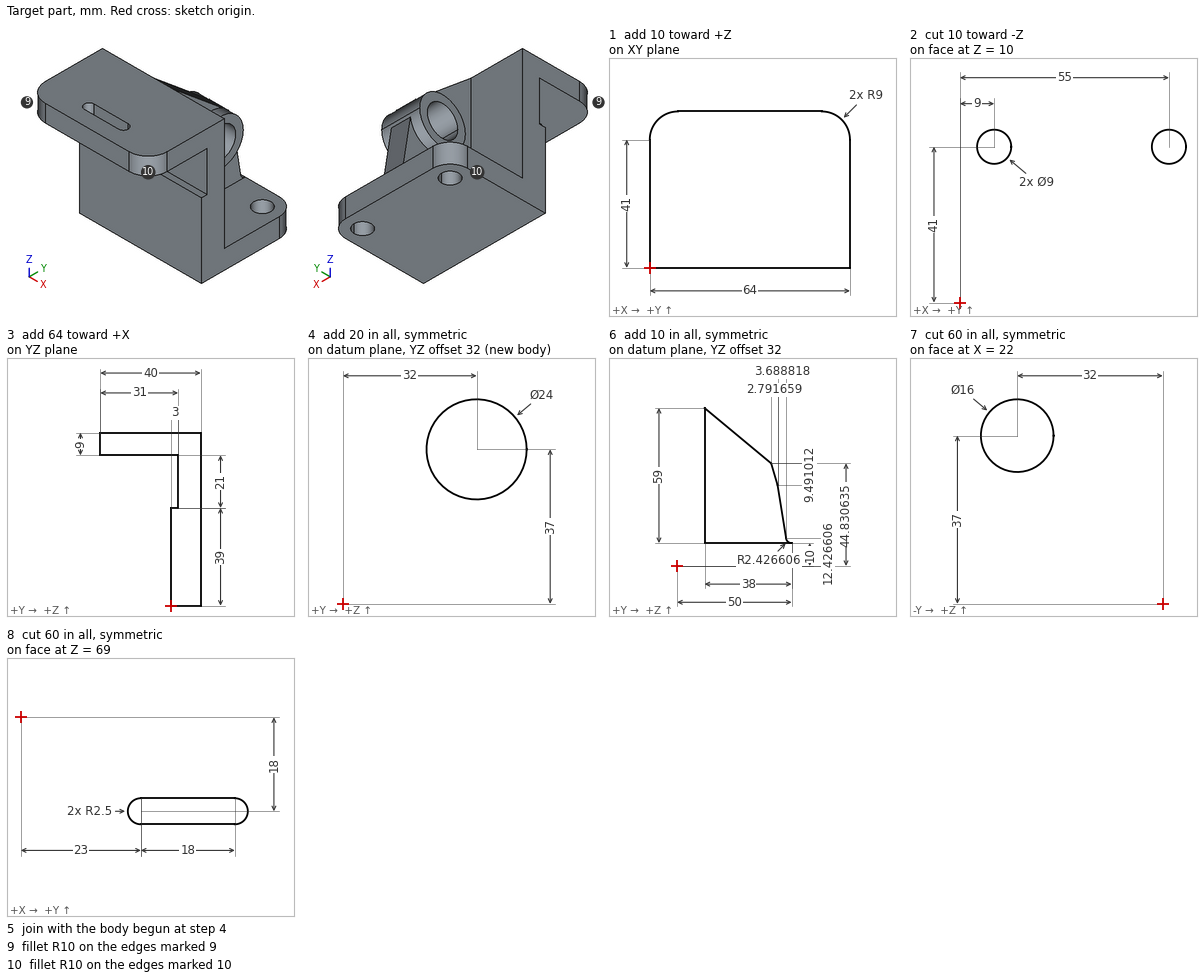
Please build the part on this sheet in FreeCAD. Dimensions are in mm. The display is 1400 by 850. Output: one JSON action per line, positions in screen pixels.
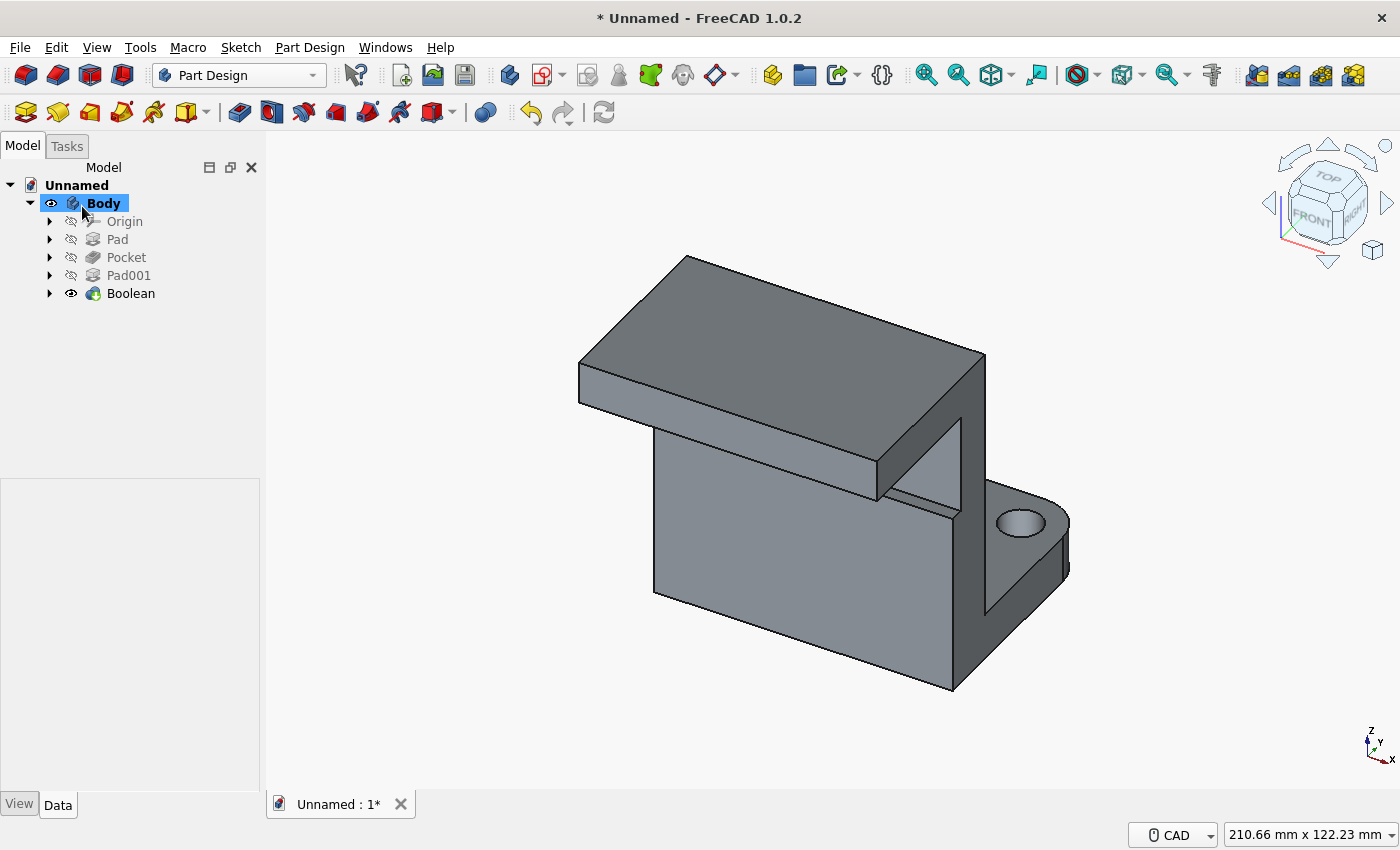
{"action": "left_click", "coordinate": [50, 221]}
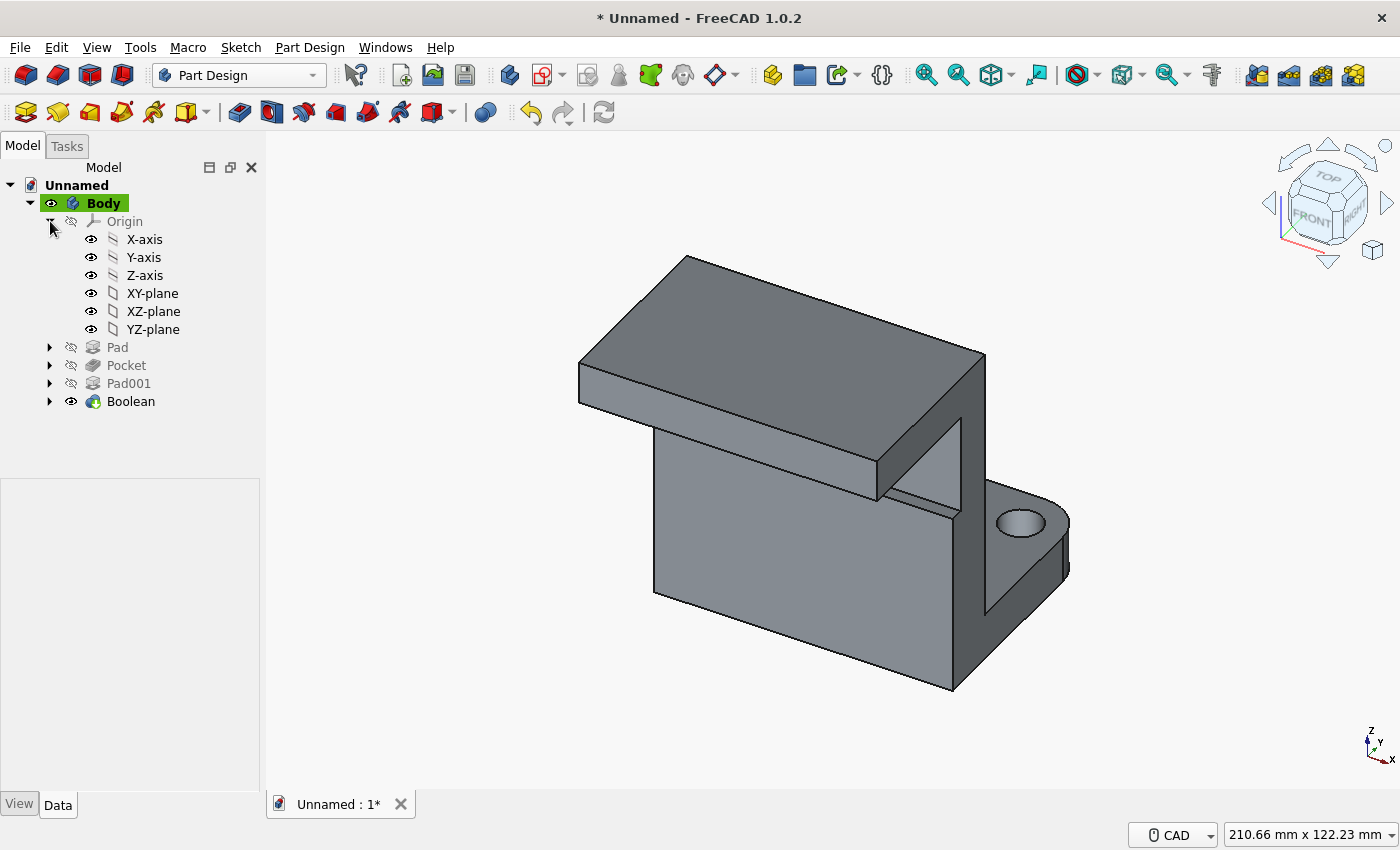
{"action": "left_click", "coordinate": [136, 329]}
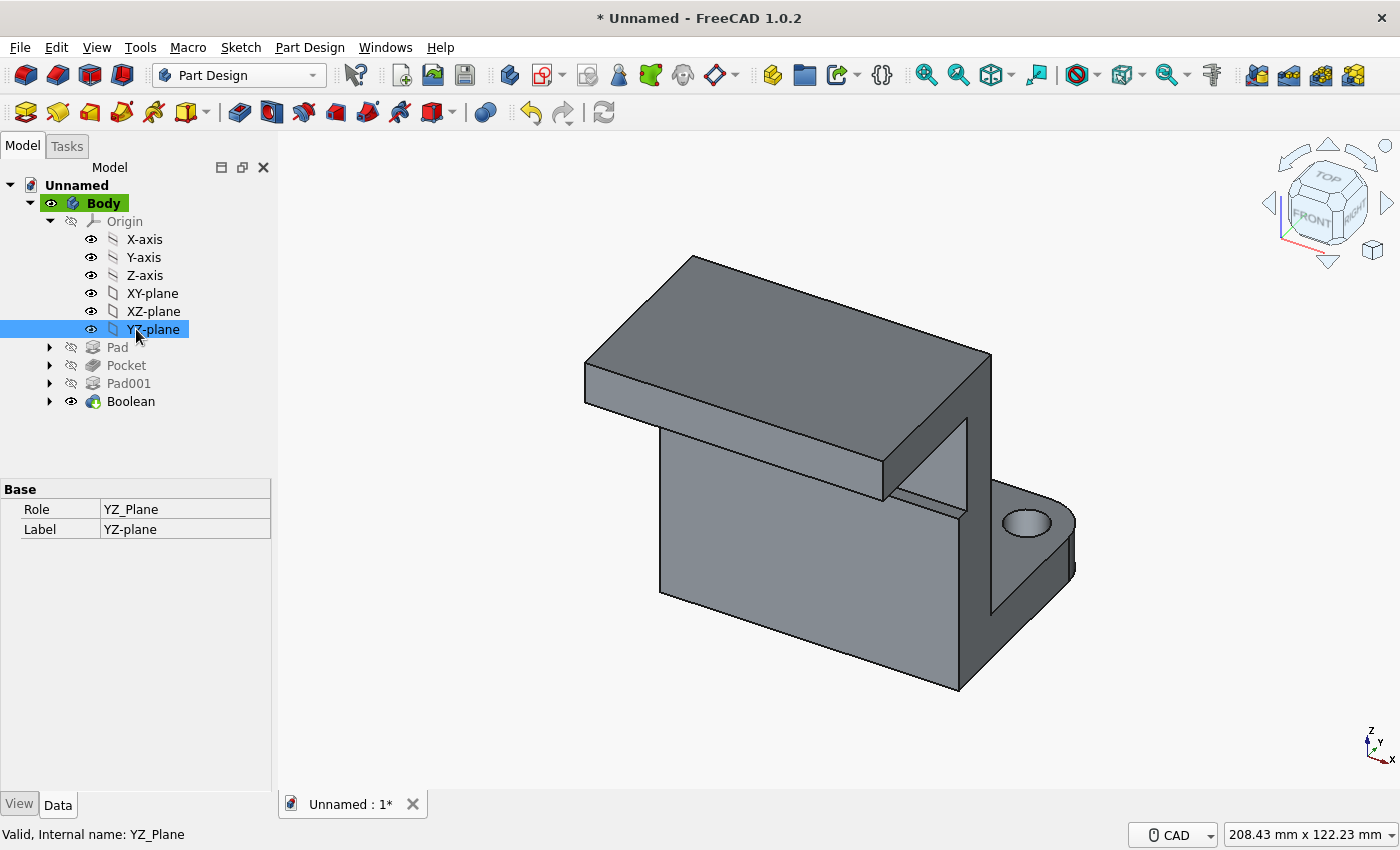
{"action": "left_click", "coordinate": [716, 76]}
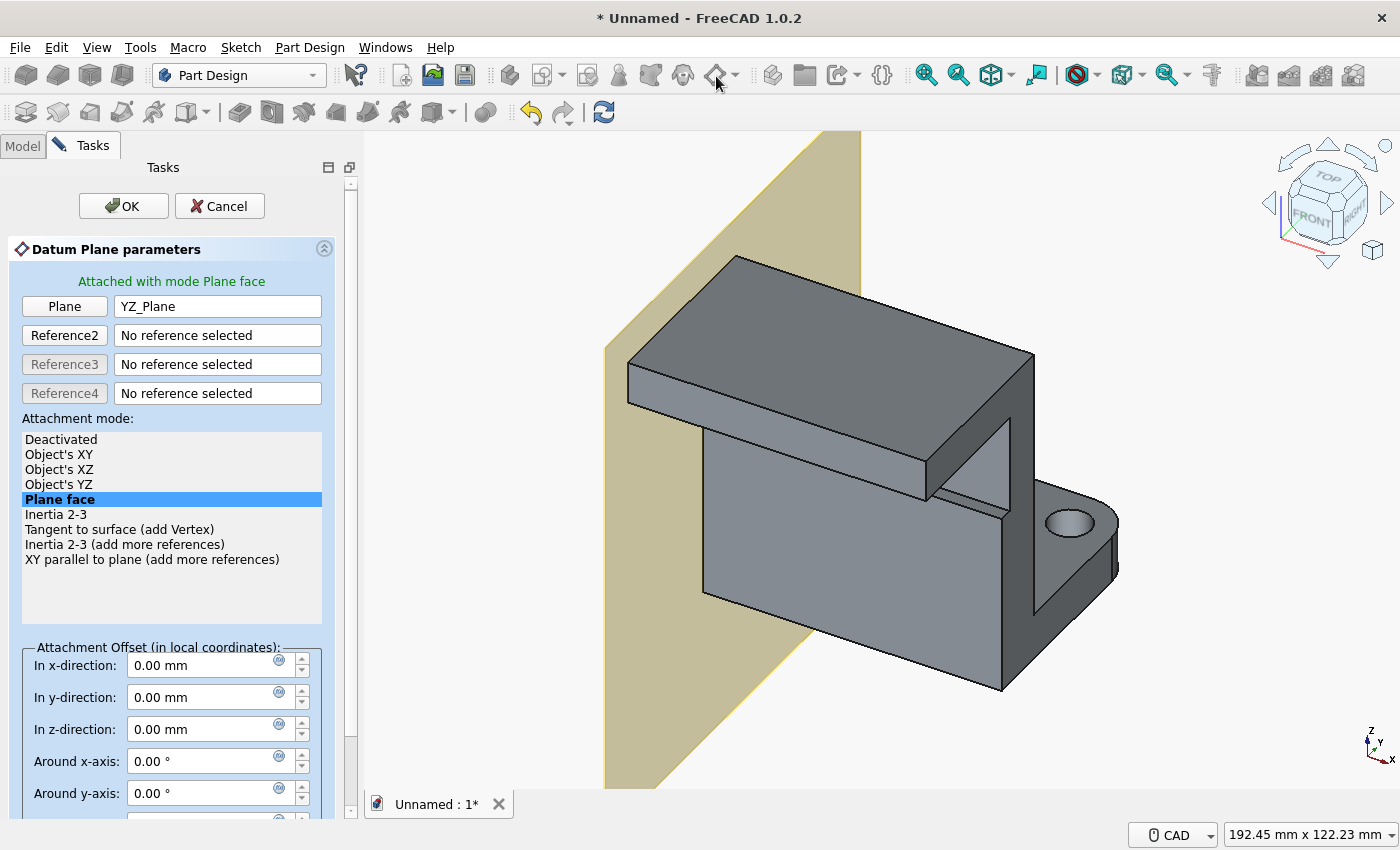
{"action": "triple_click", "coordinate": [210, 729]}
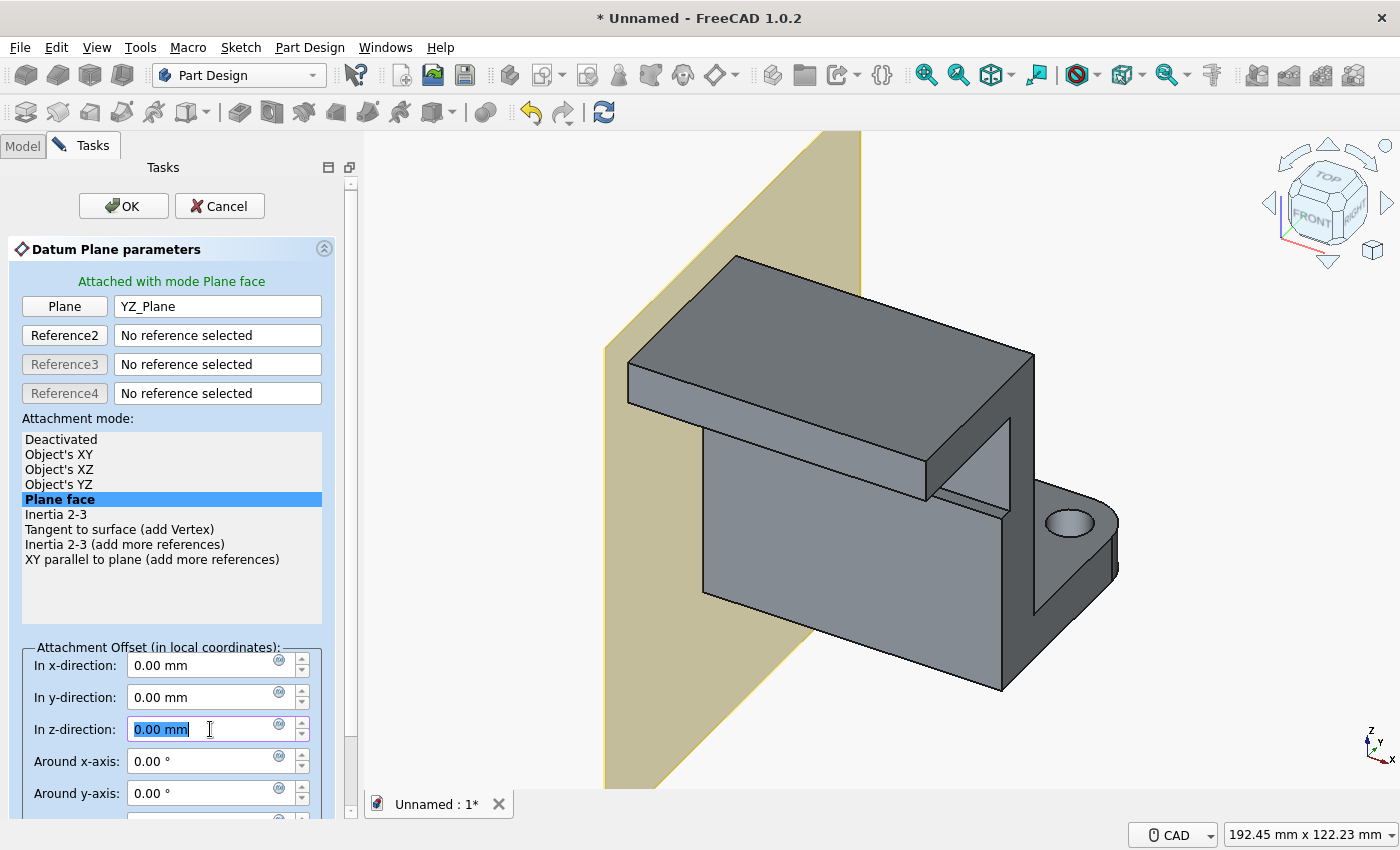
{"action": "type", "text": "32"}
{"action": "key", "text": "Tab"}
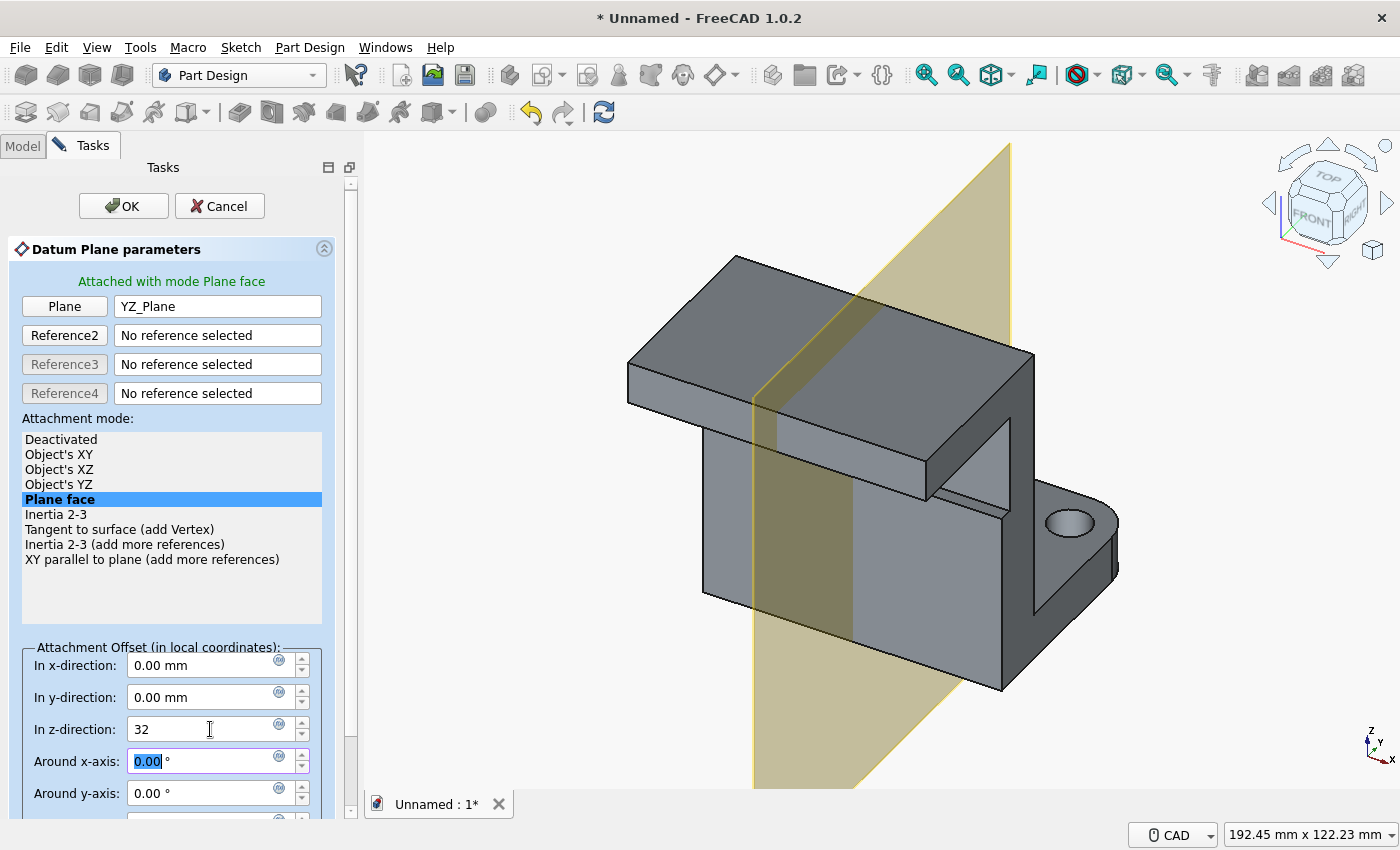
{"action": "left_click", "coordinate": [124, 206]}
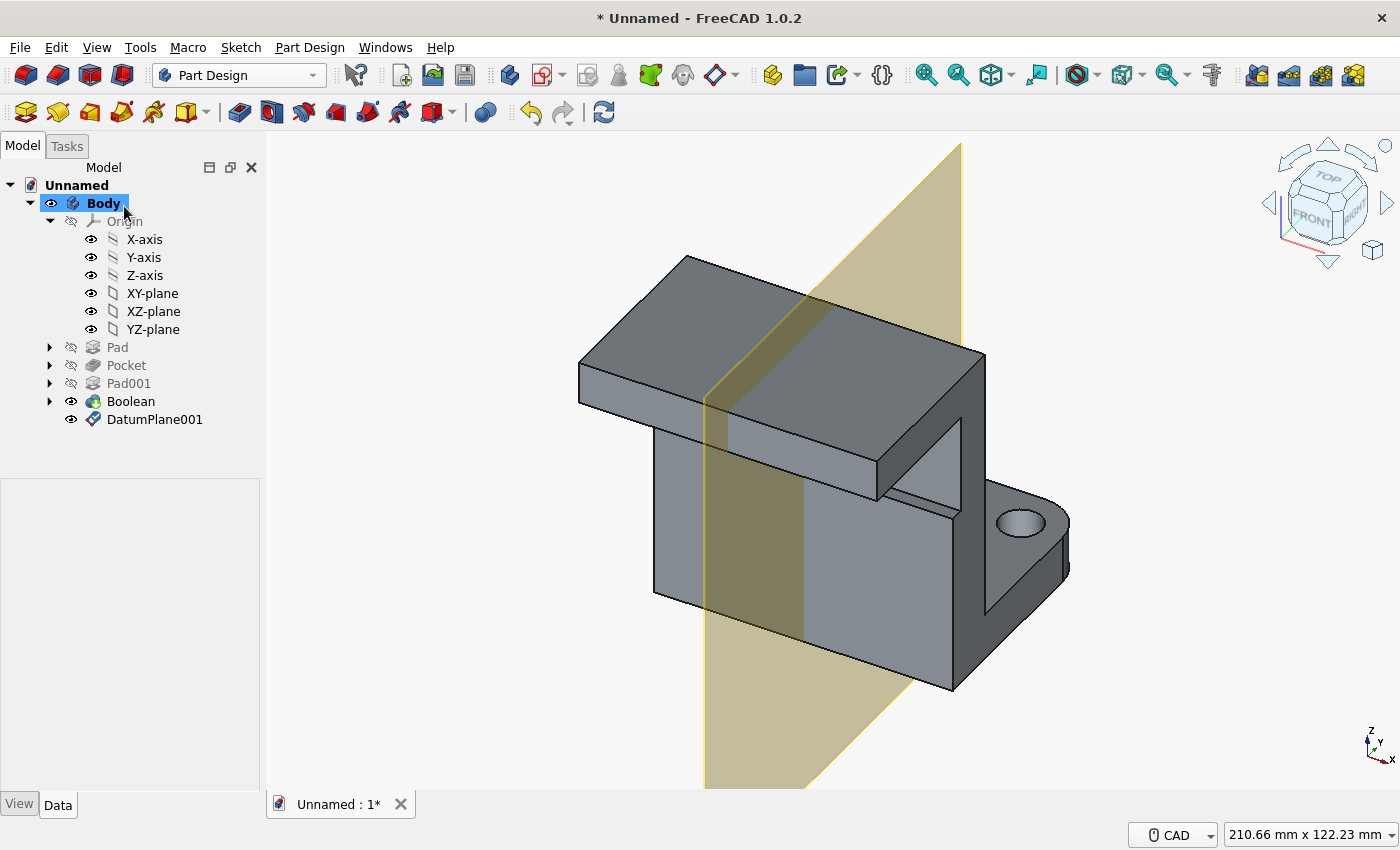
{"action": "left_click", "coordinate": [116, 419]}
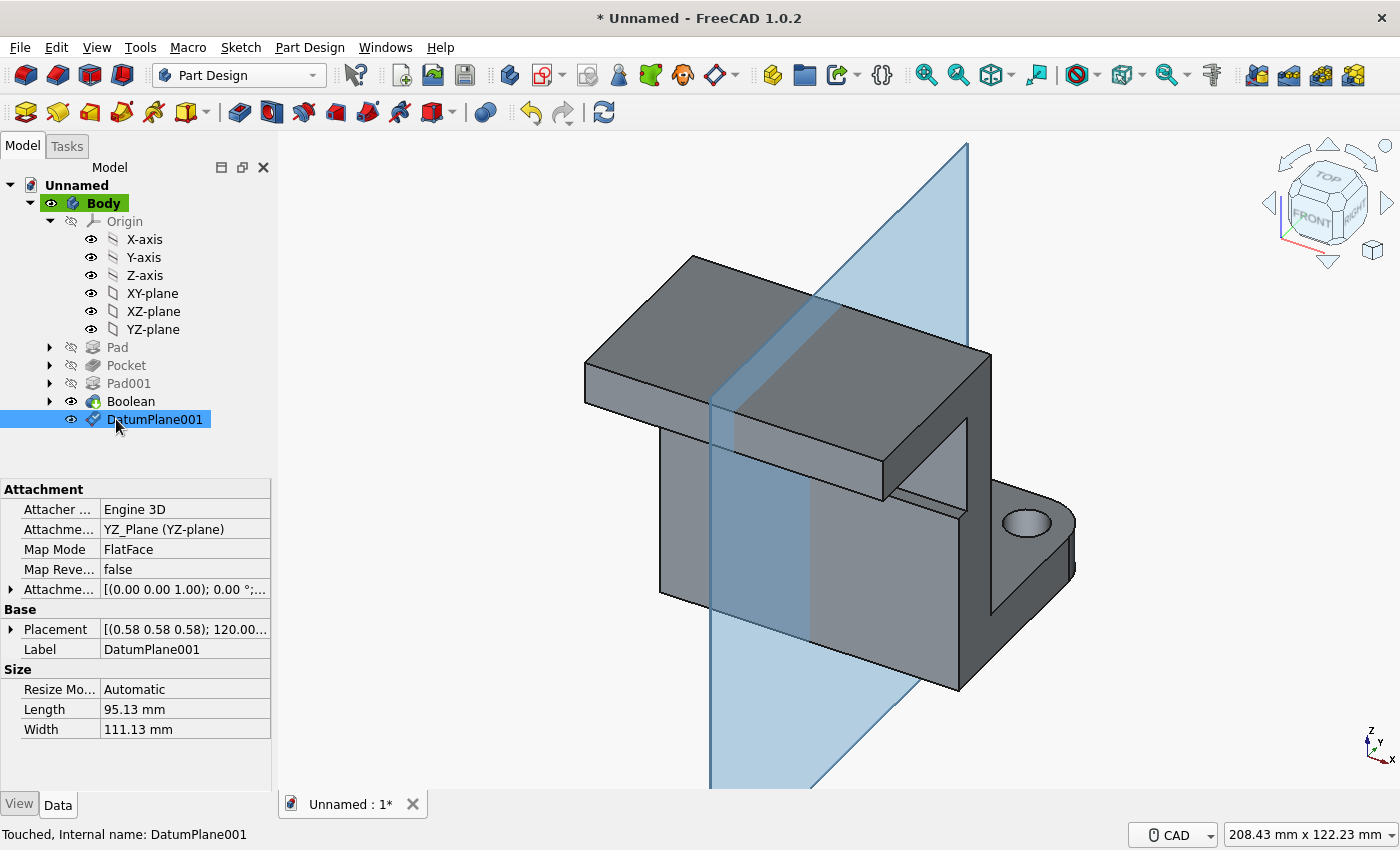
{"action": "left_click", "coordinate": [542, 76]}